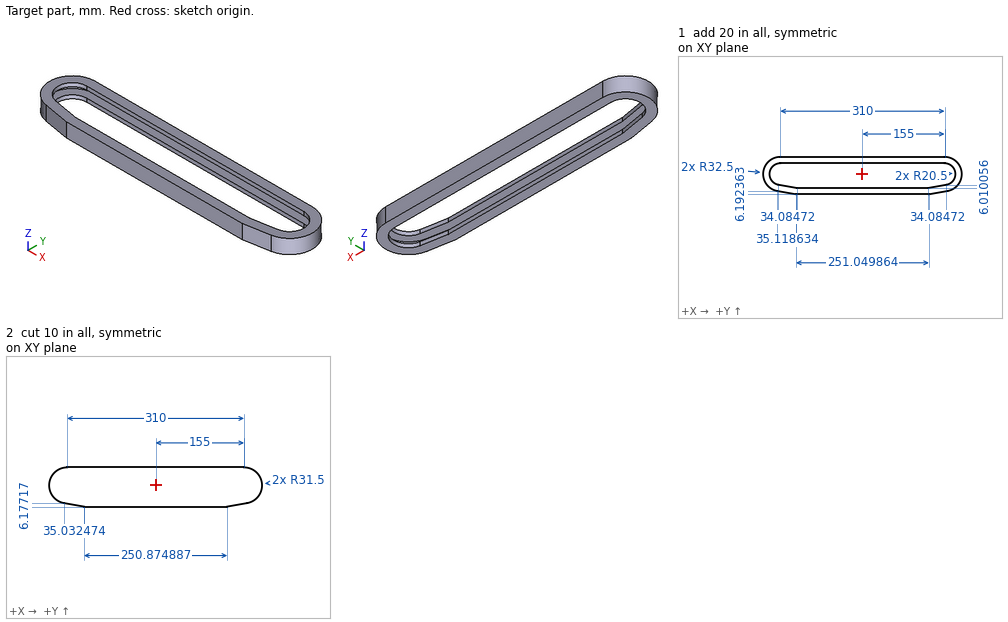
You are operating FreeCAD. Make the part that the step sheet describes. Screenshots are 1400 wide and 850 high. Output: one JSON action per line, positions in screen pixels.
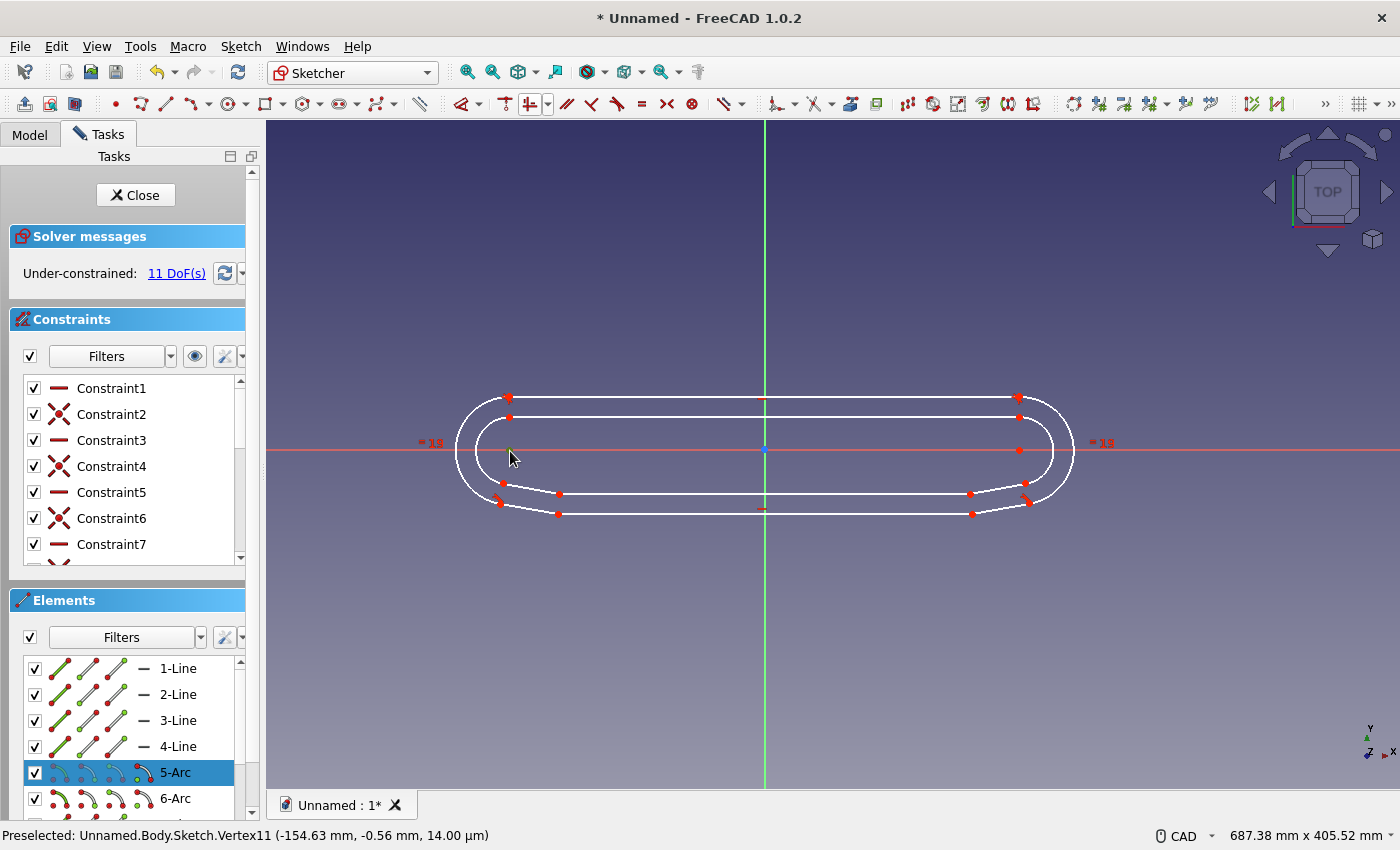
{"action": "left_click", "coordinate": [361, 450]}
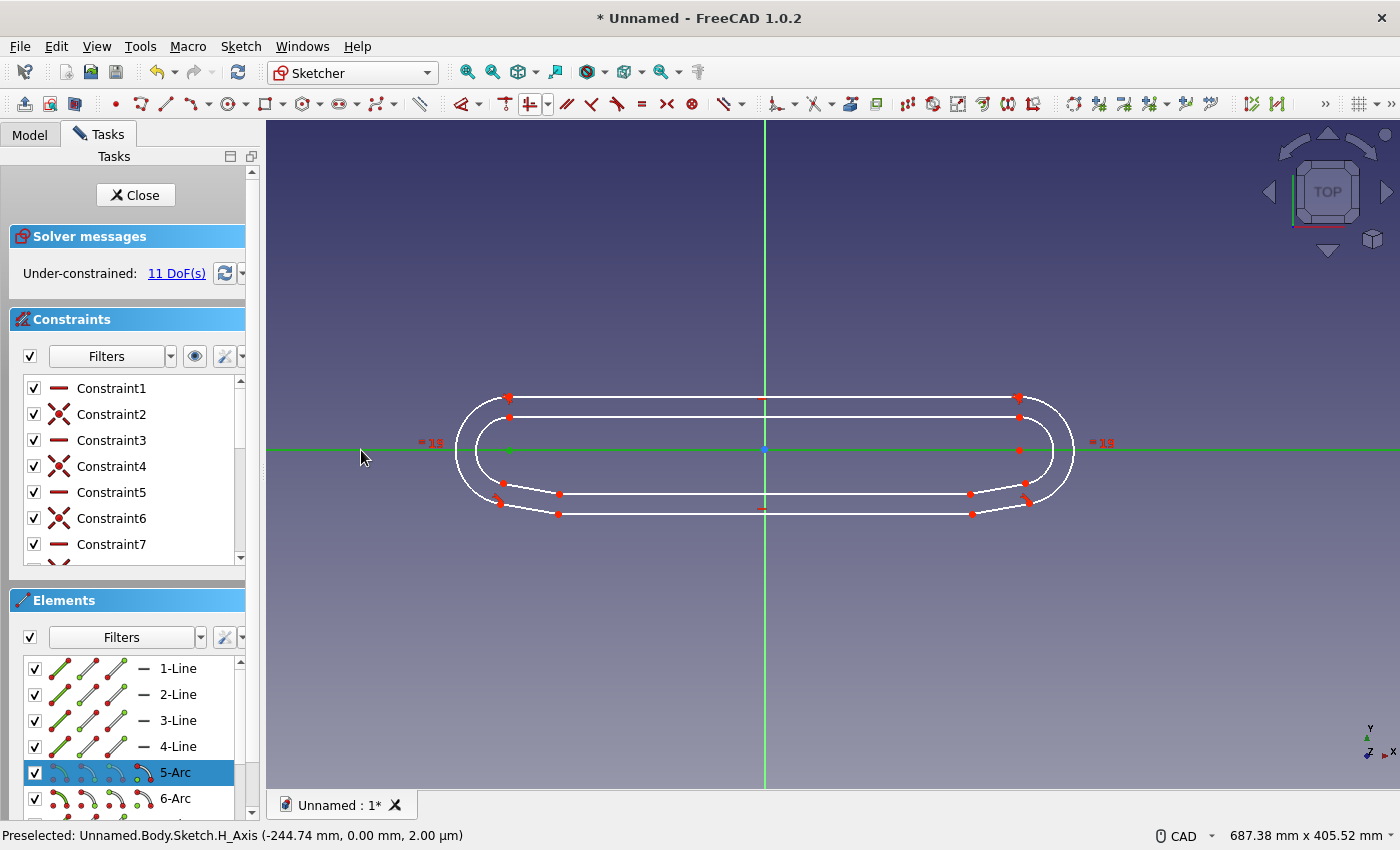
{"action": "key", "text": "c"}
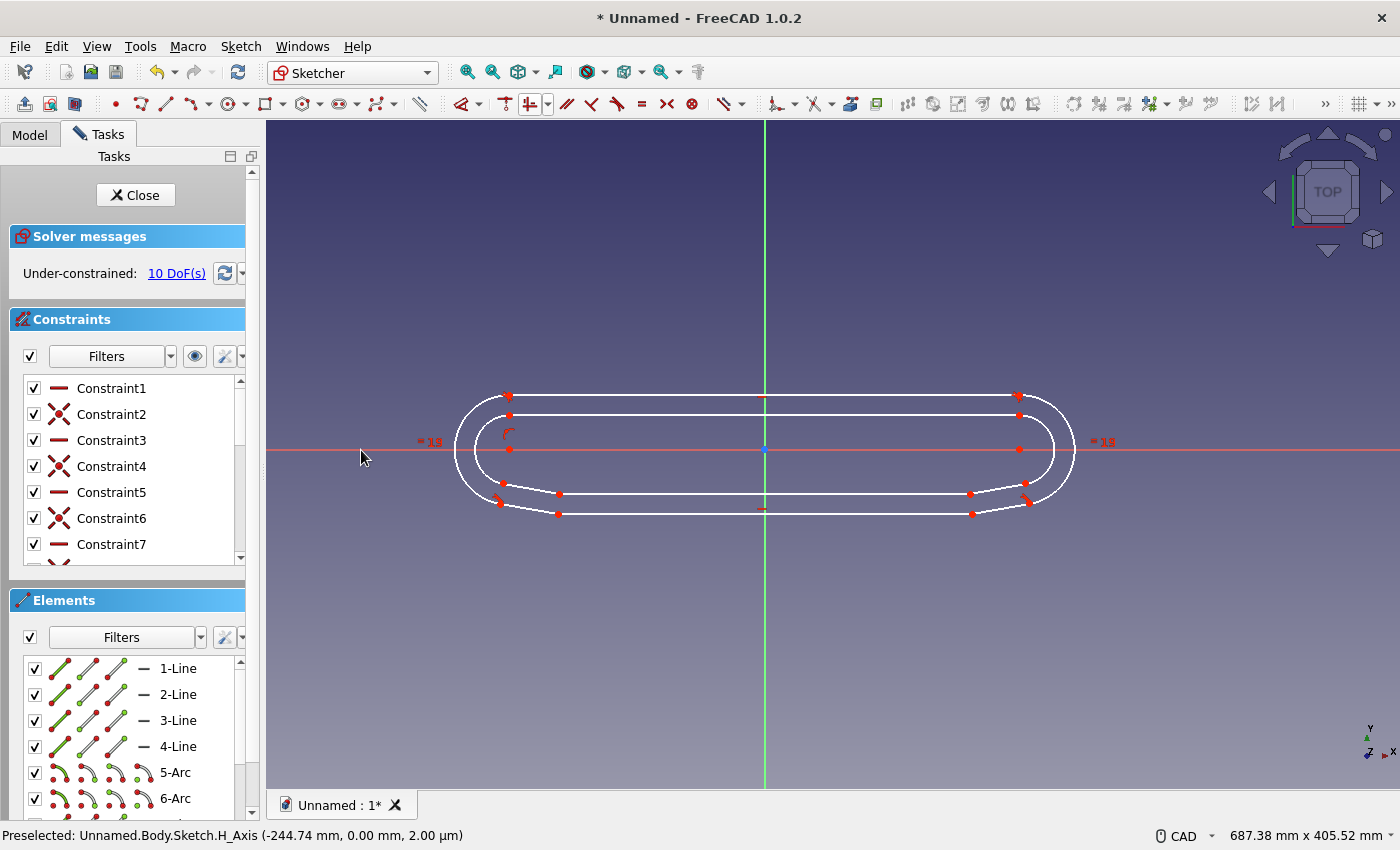
{"action": "left_click", "coordinate": [467, 415]}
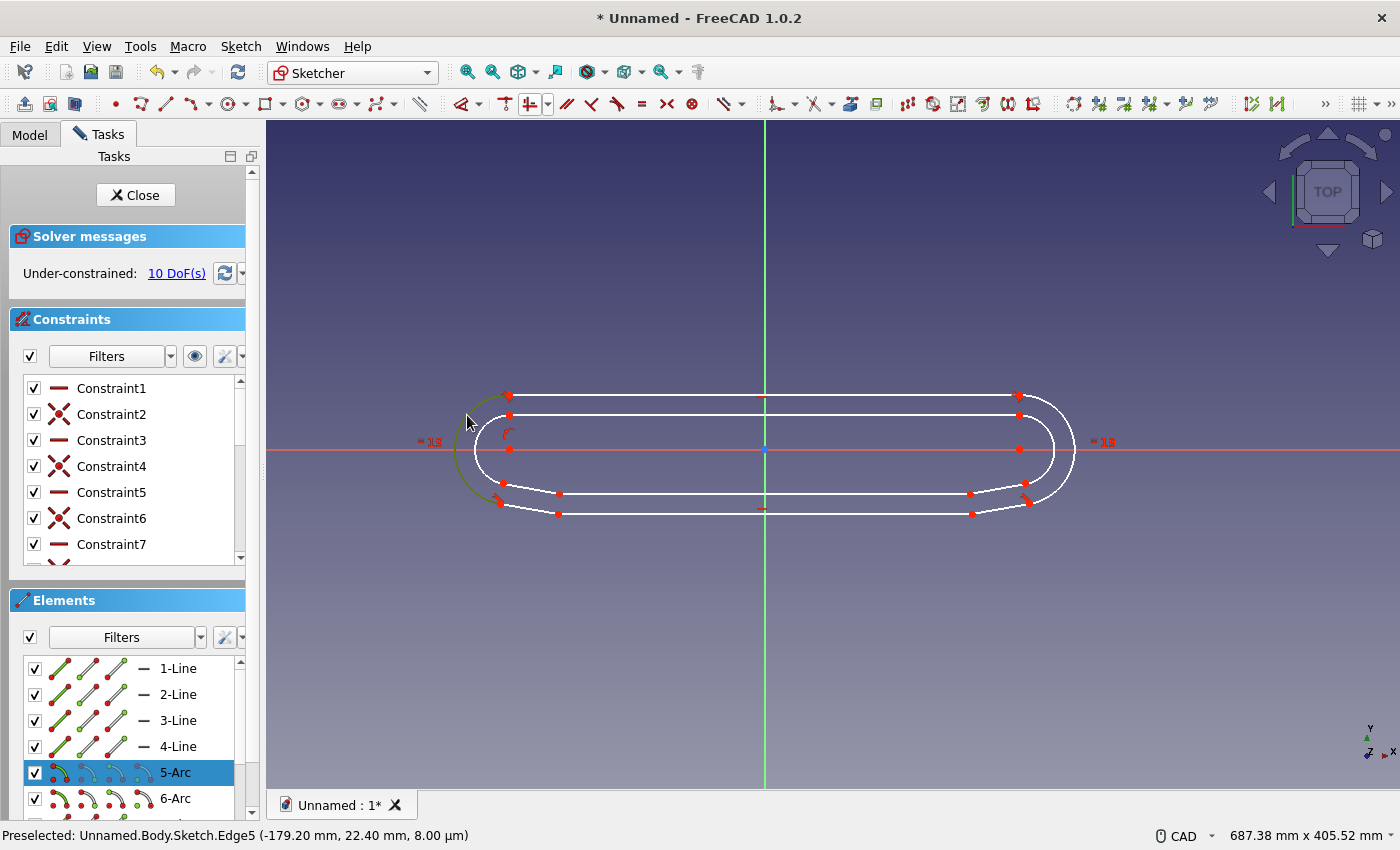
{"action": "key", "text": "k r"}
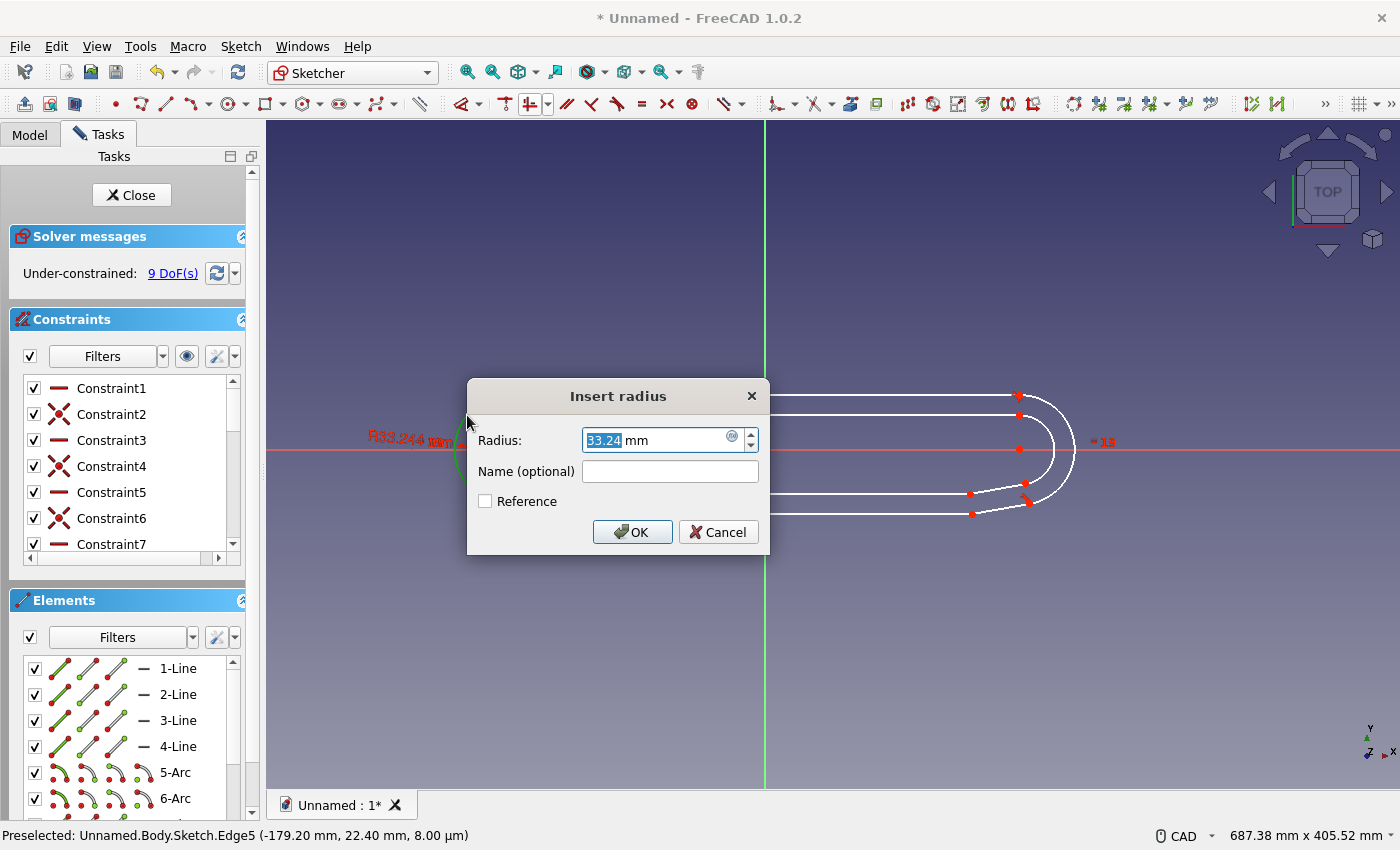
{"action": "type", "text": "32.5"}
{"action": "key", "text": "Return"}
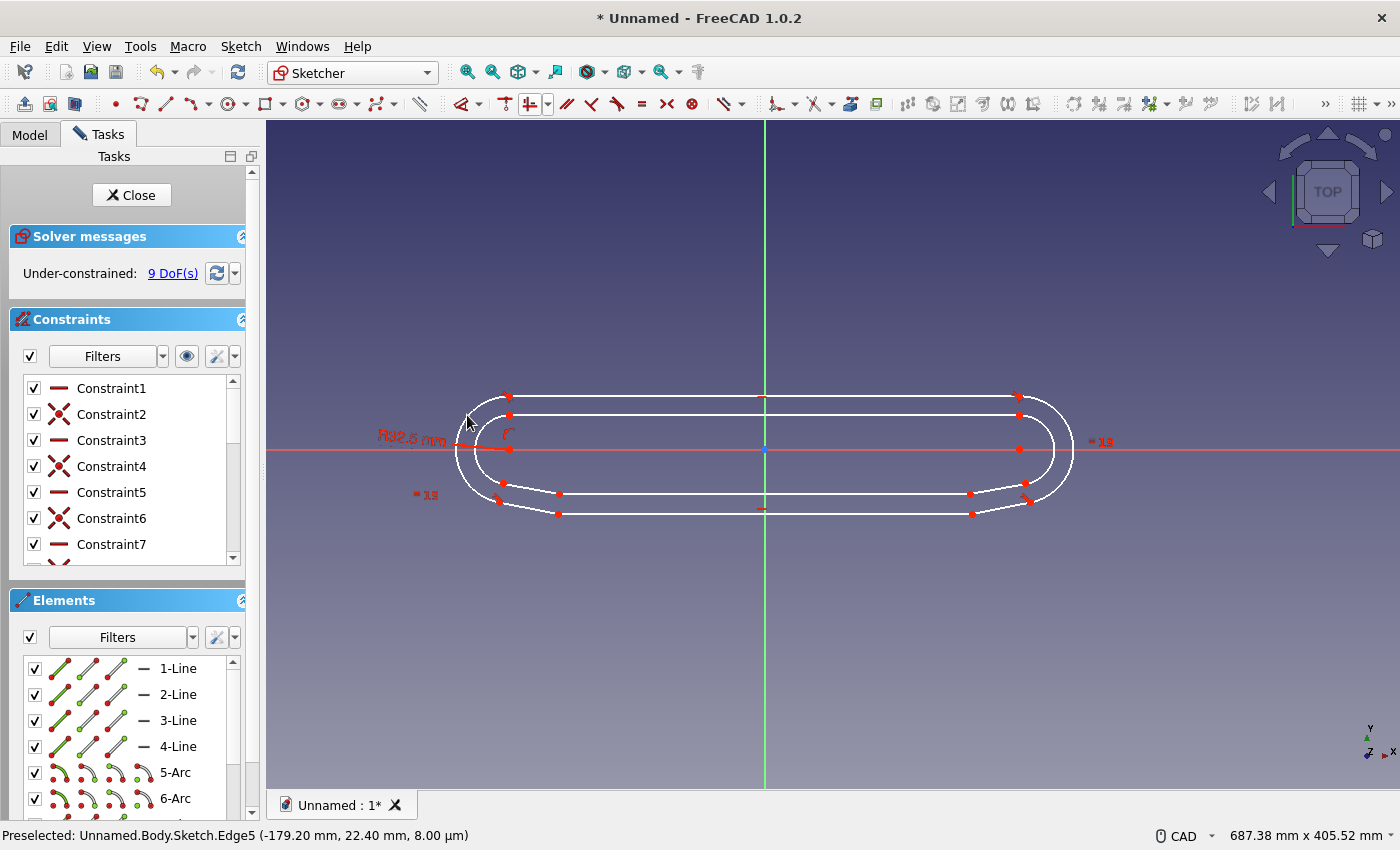
{"action": "left_click", "coordinate": [1050, 467]}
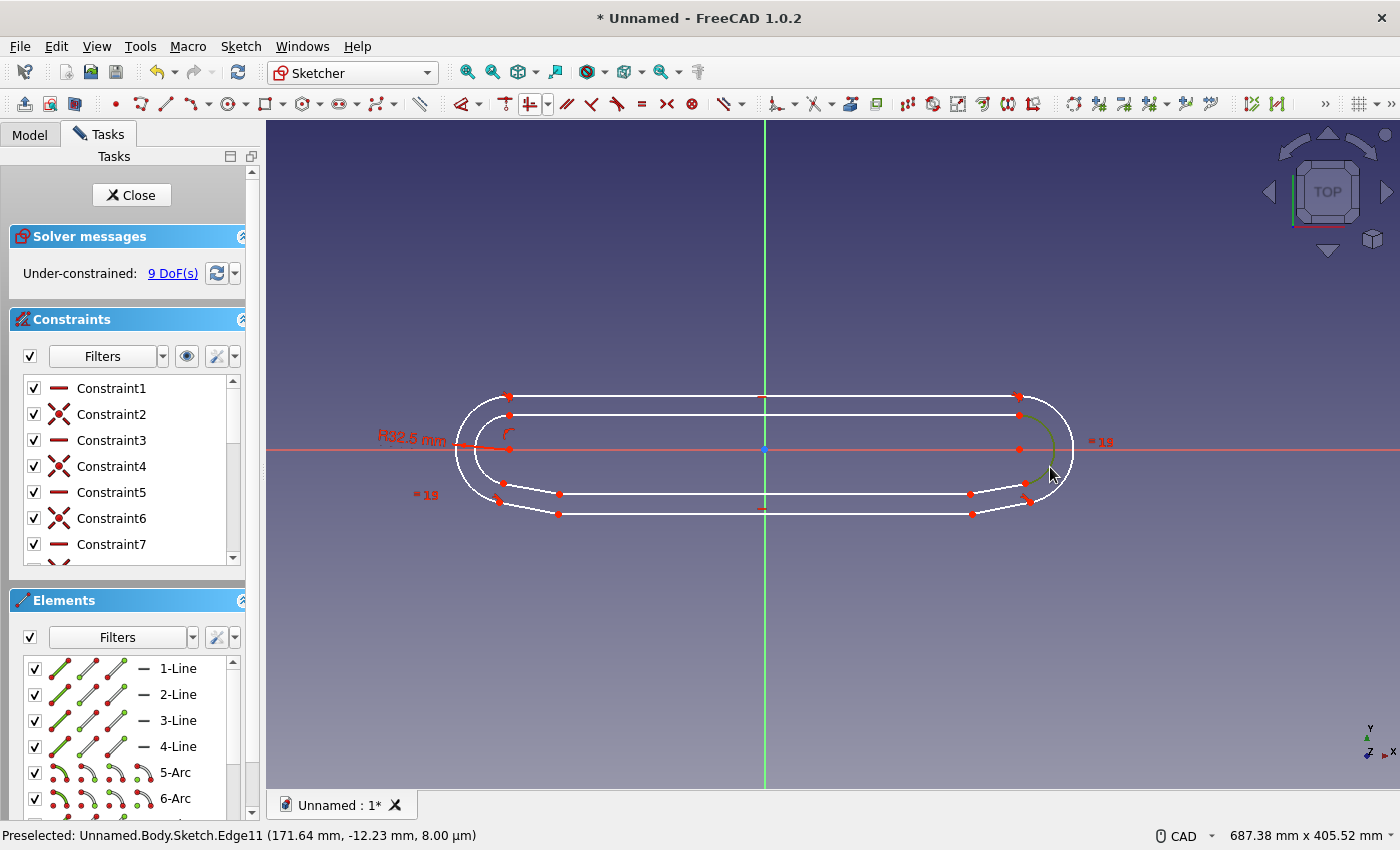
{"action": "key", "text": "k r"}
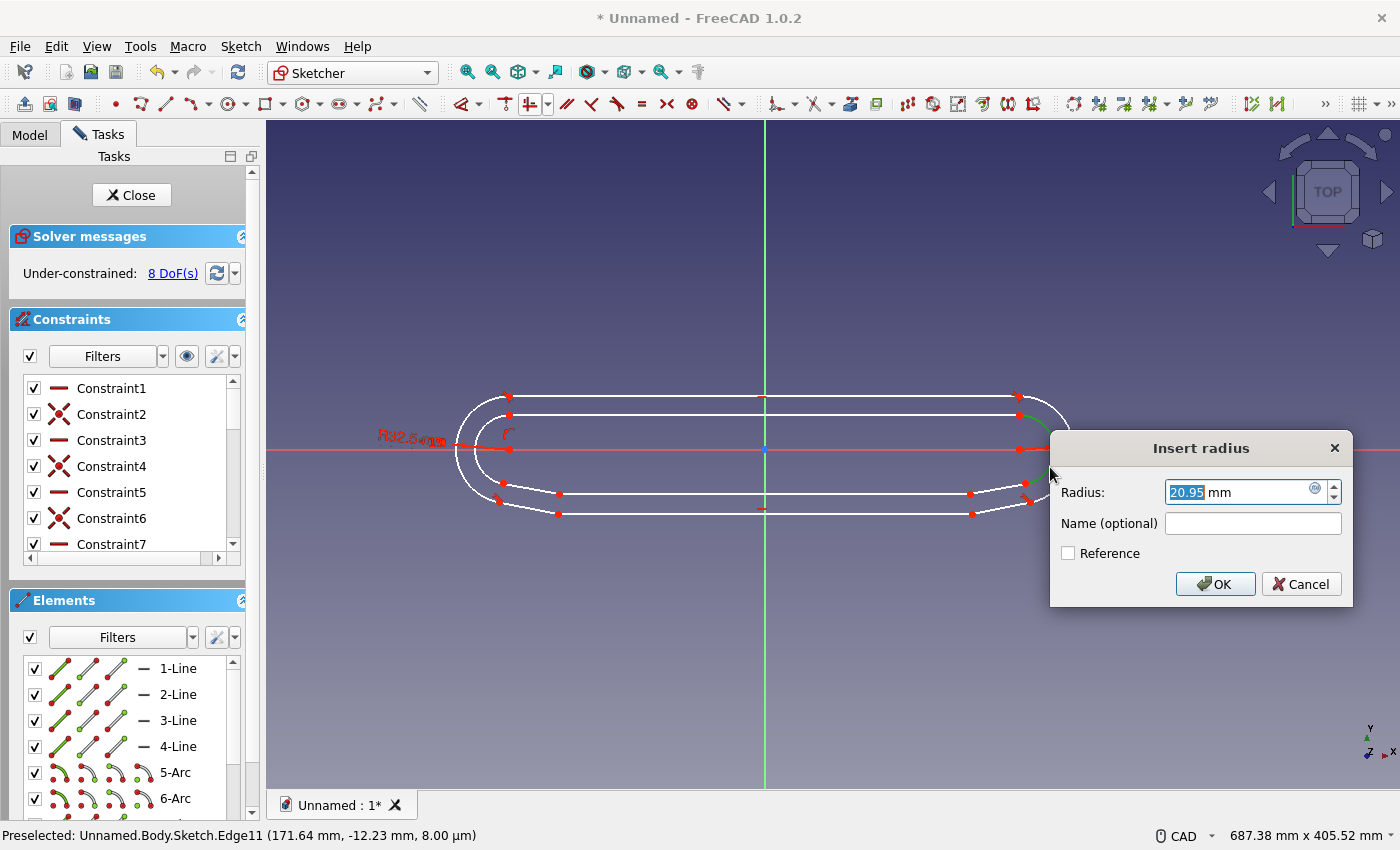
{"action": "type", "text": "20.5"}
{"action": "key", "text": "Return"}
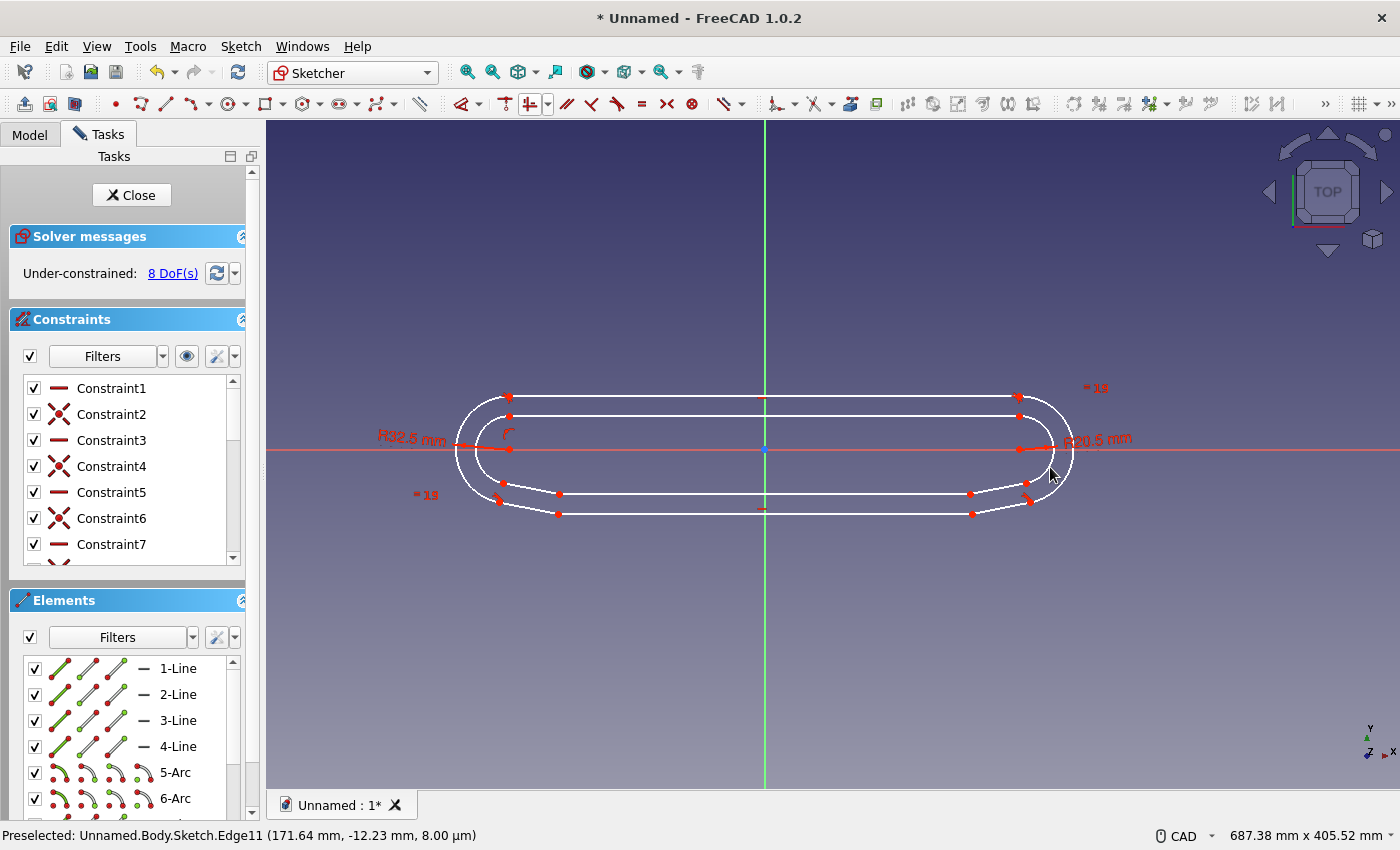
{"action": "left_click", "coordinate": [867, 396]}